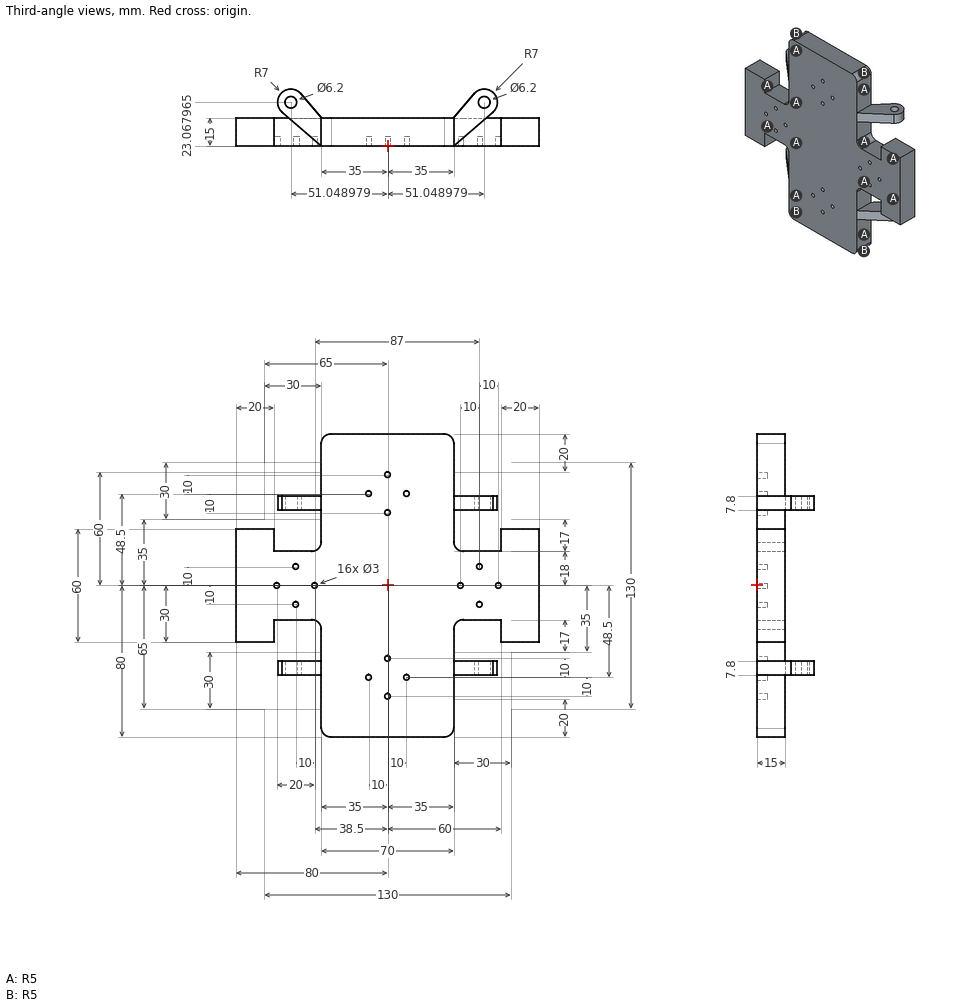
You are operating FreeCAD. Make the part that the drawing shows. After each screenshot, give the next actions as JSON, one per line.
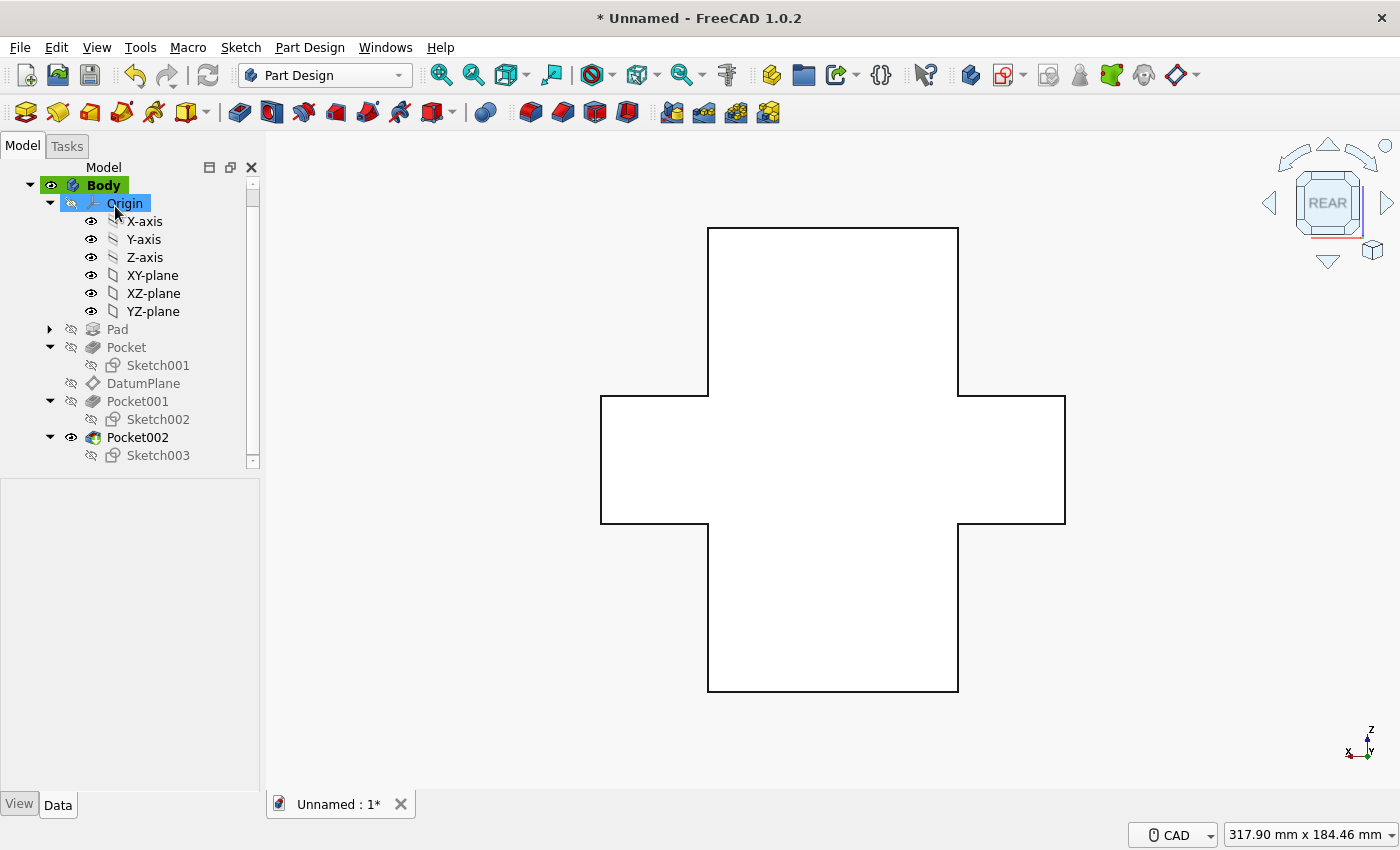
{"action": "key", "text": "0"}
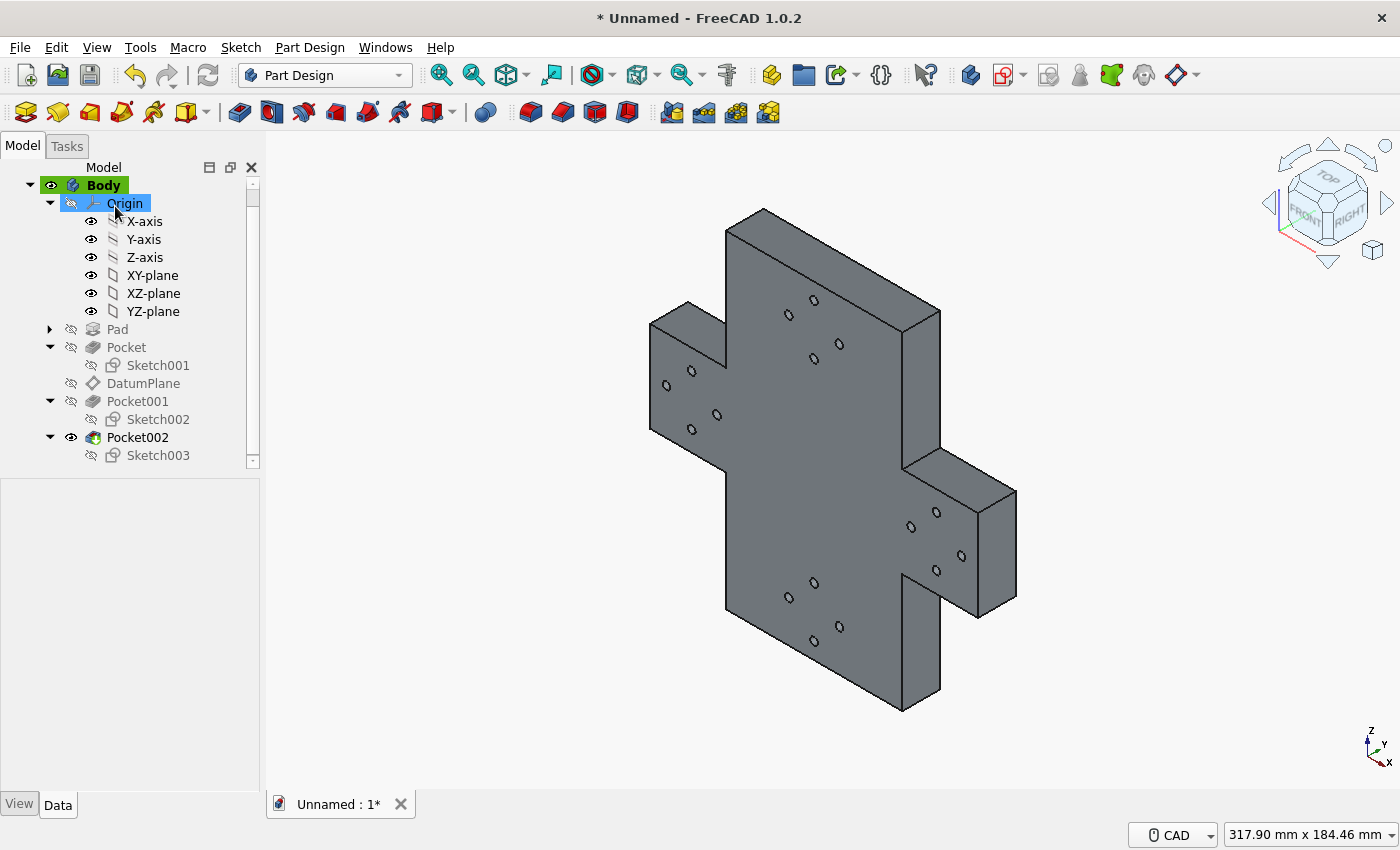
{"action": "left_click", "coordinate": [997, 501]}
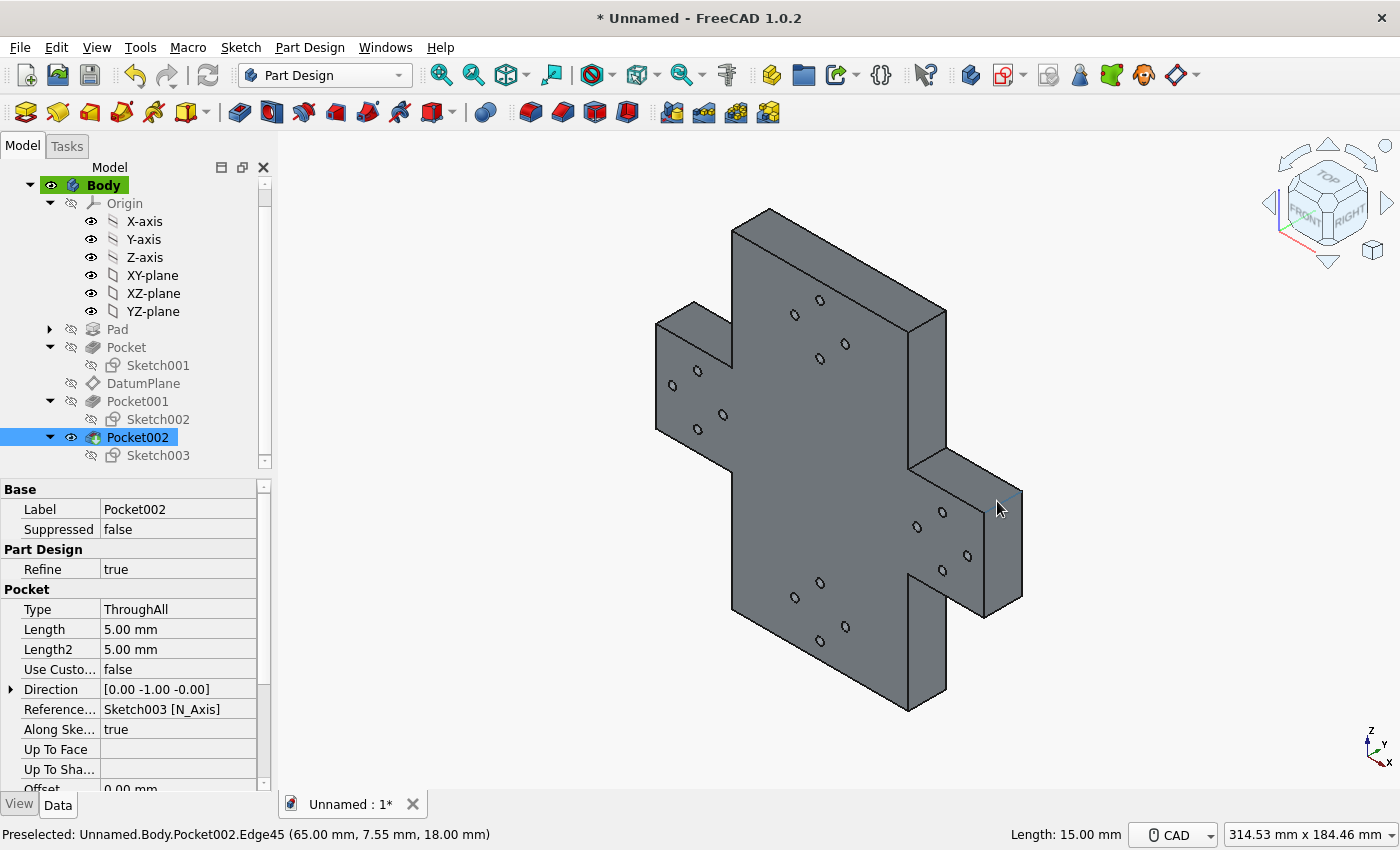
{"action": "left_click", "coordinate": [927, 321], "text": "ctrl"}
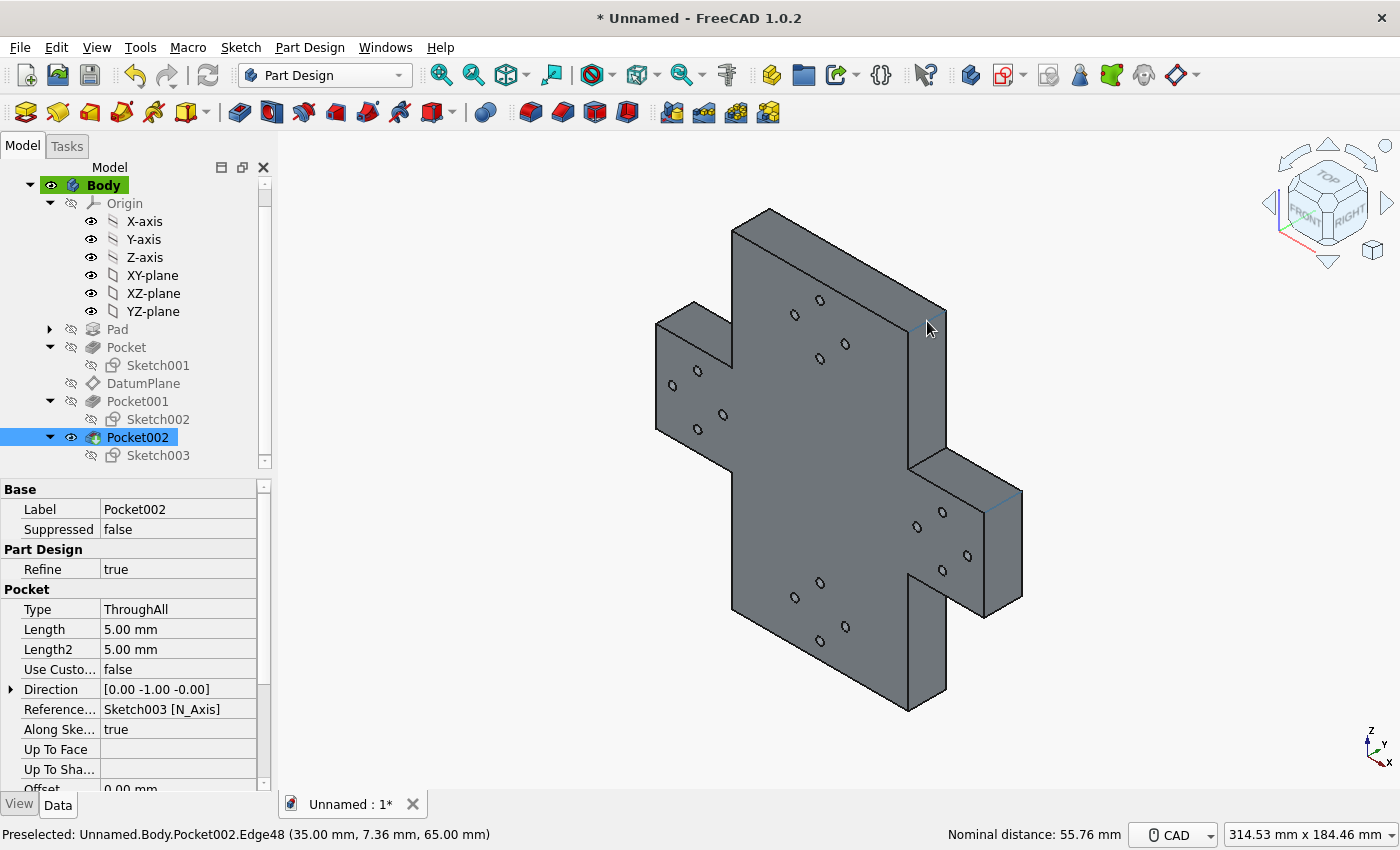
{"action": "key", "text": "2"}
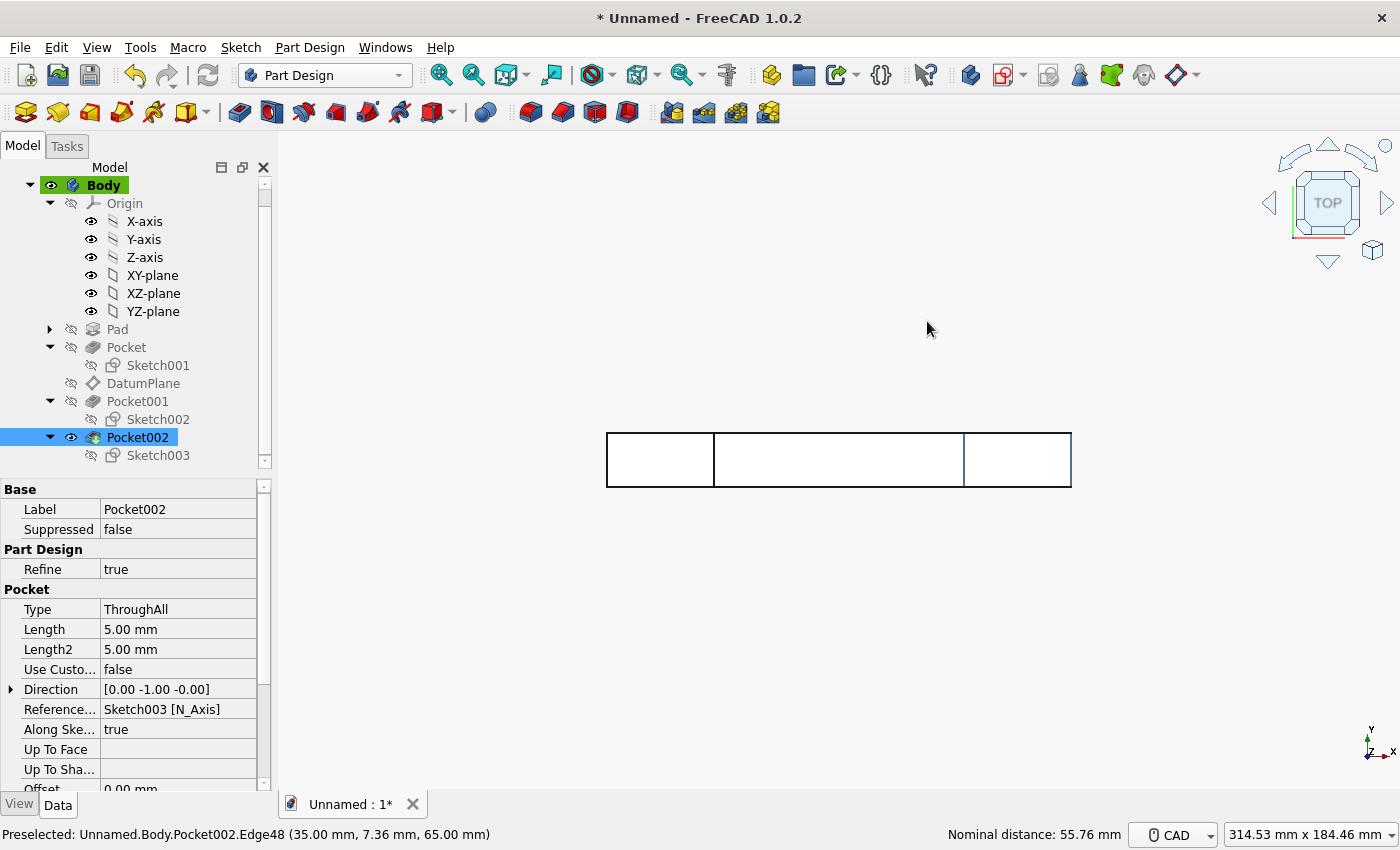
{"action": "left_click", "coordinate": [442, 76]}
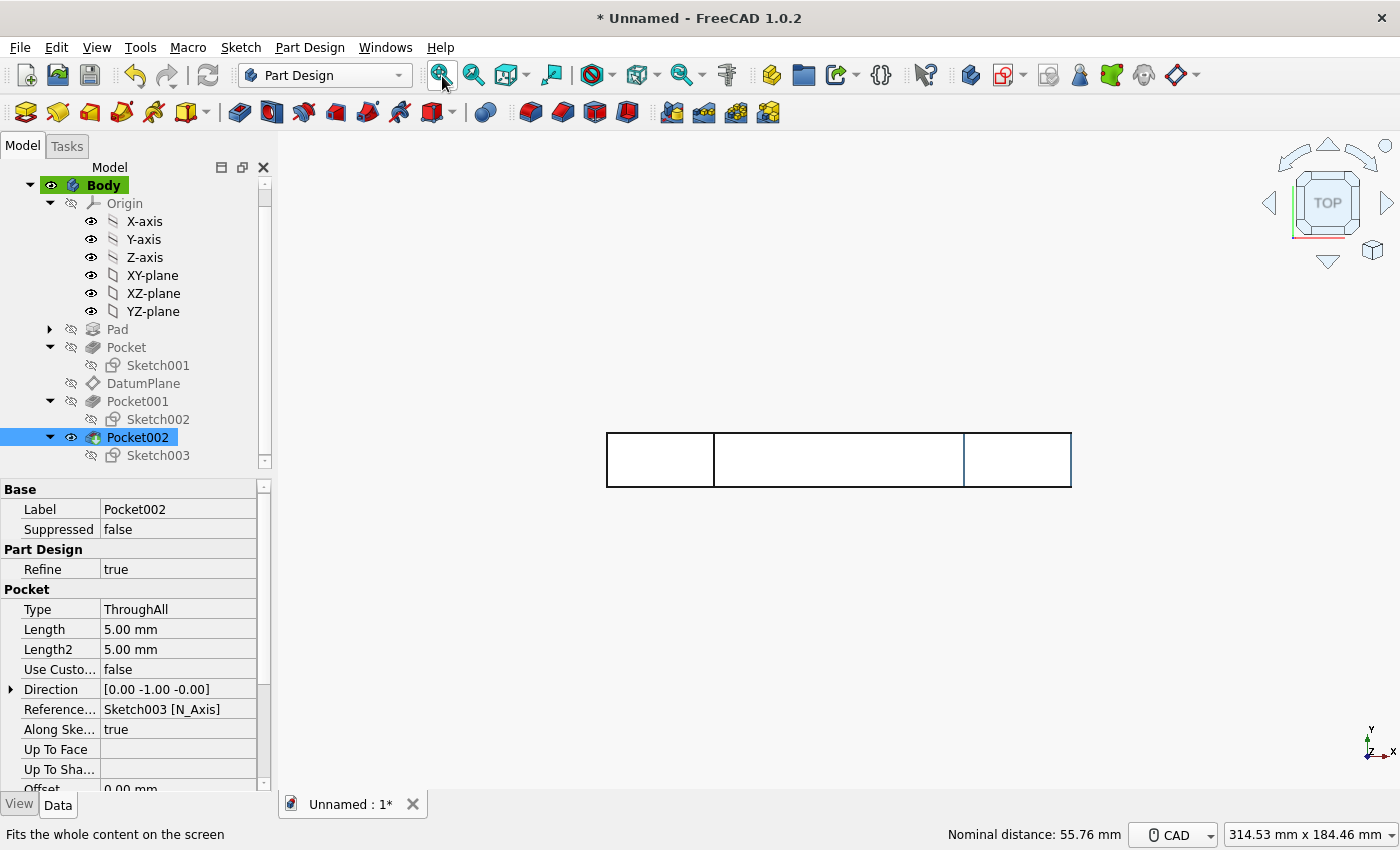
{"action": "left_click", "coordinate": [607, 459], "text": "ctrl"}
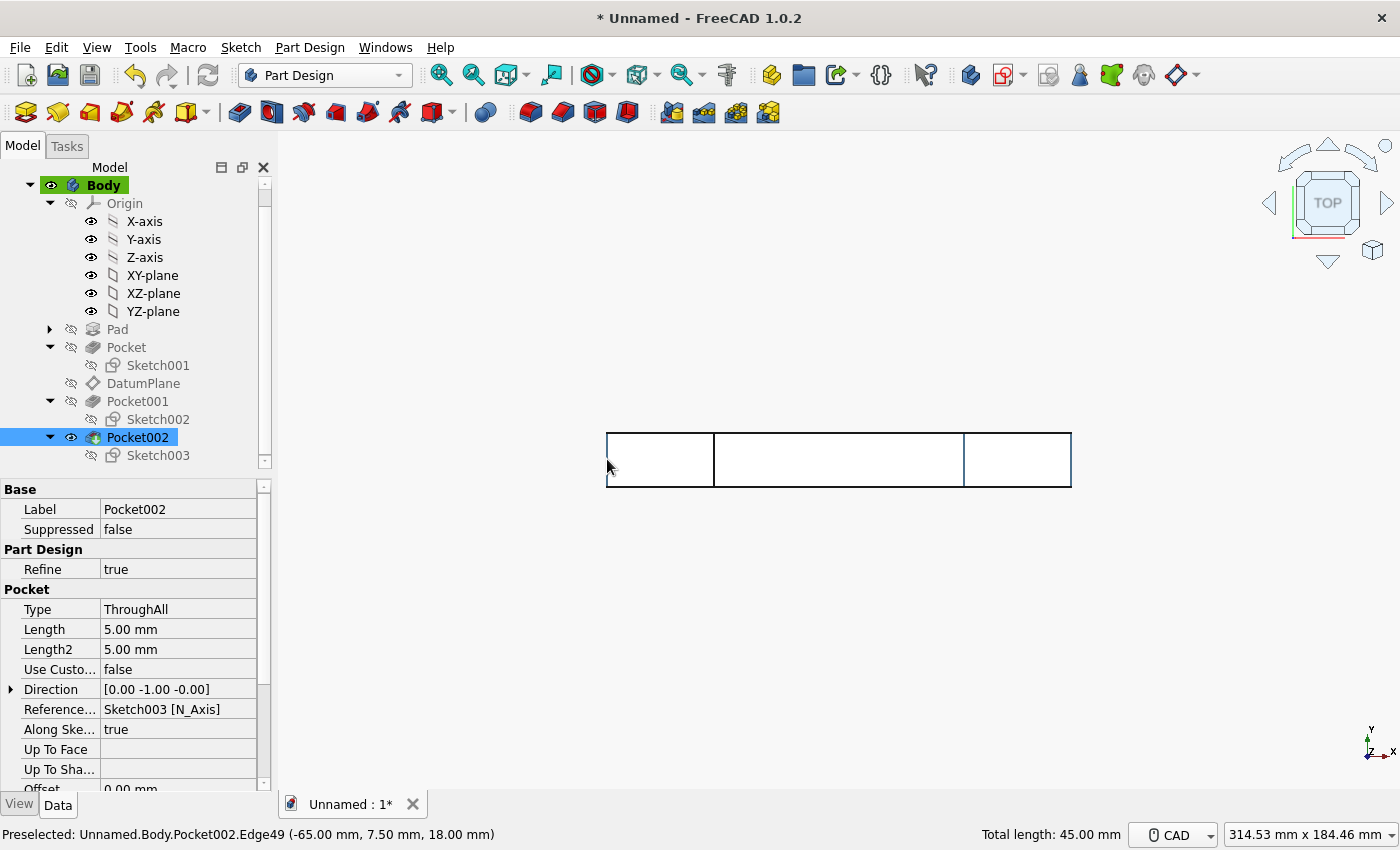
{"action": "left_click", "coordinate": [714, 459], "text": "ctrl"}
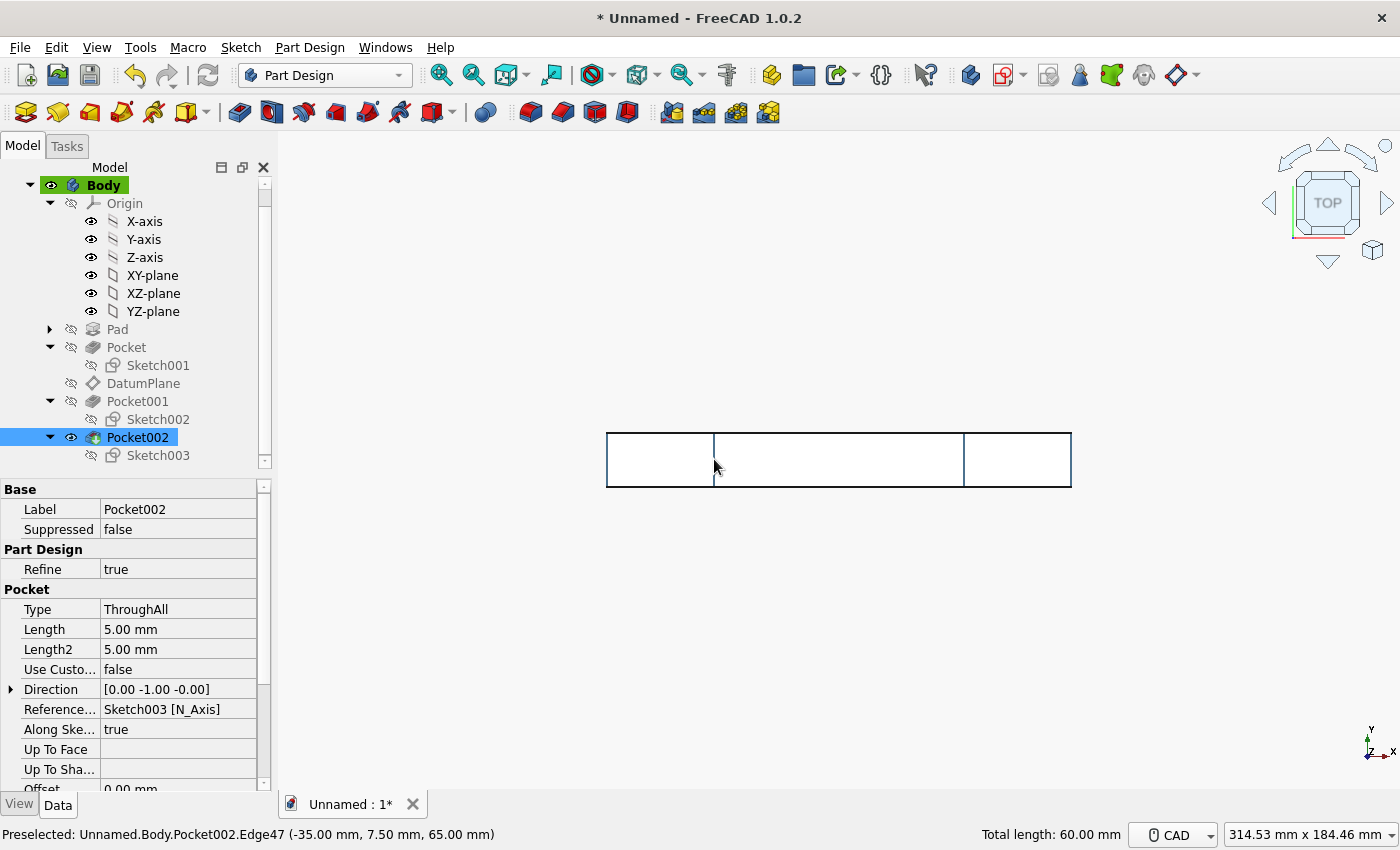
{"action": "key", "text": "1"}